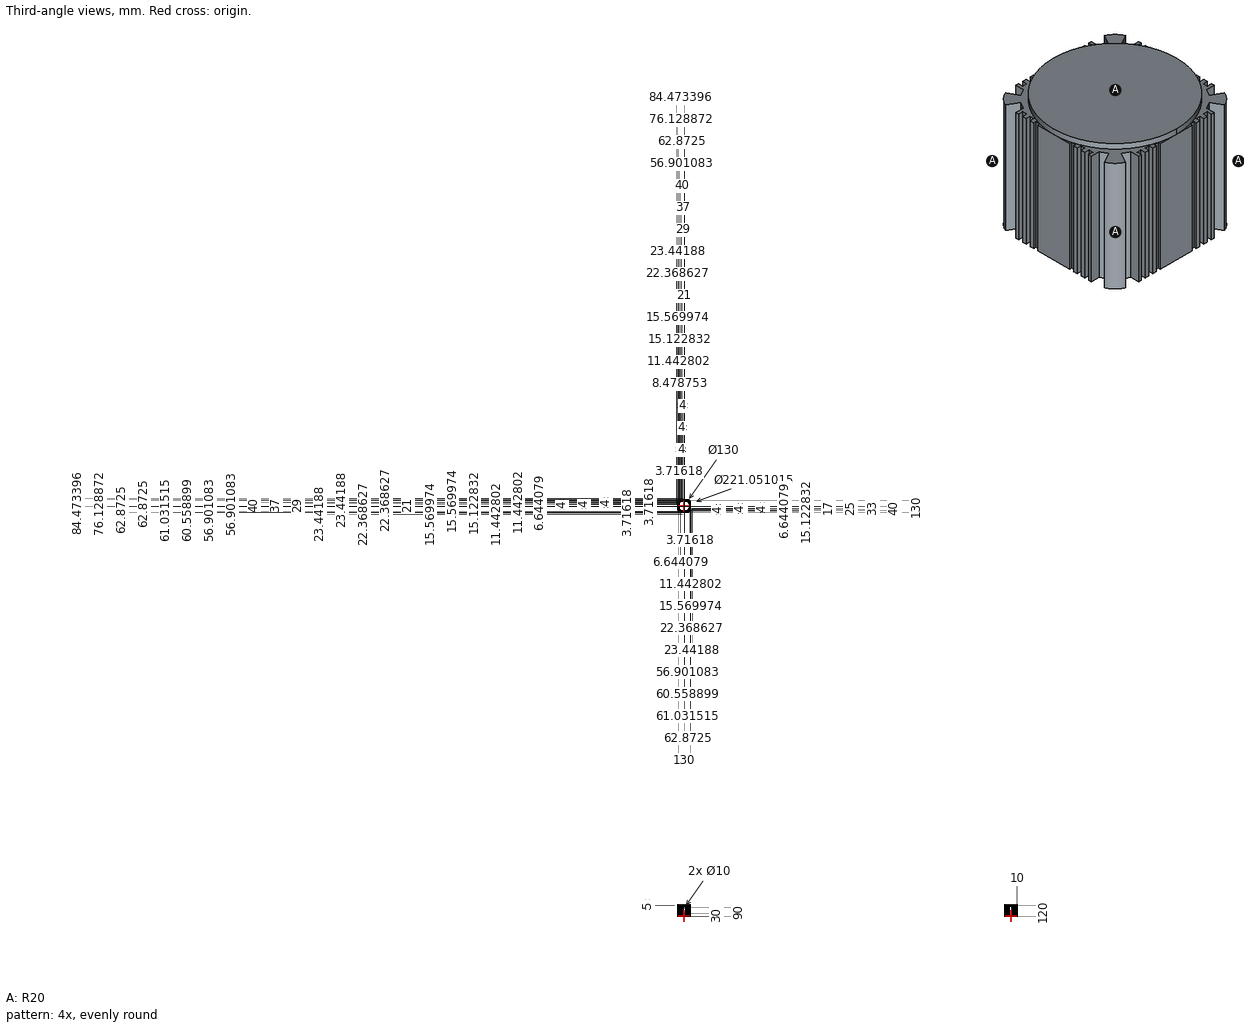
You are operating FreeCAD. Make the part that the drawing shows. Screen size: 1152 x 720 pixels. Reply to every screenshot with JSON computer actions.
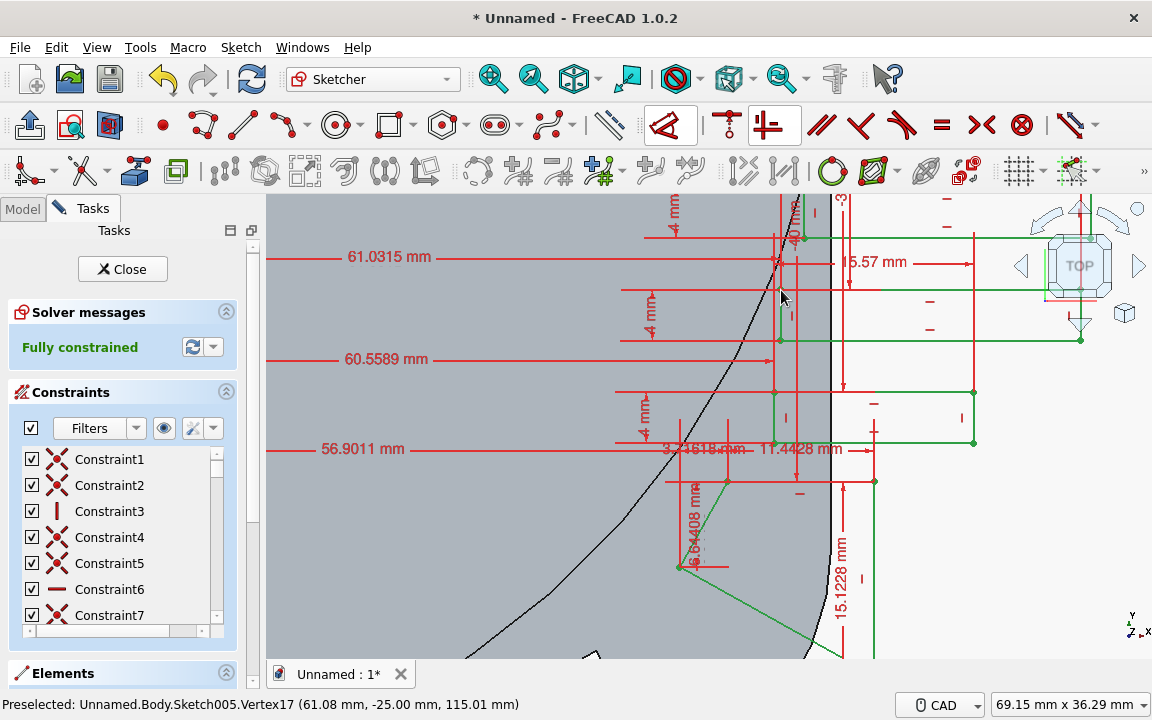
{"action": "left_click", "coordinate": [123, 269]}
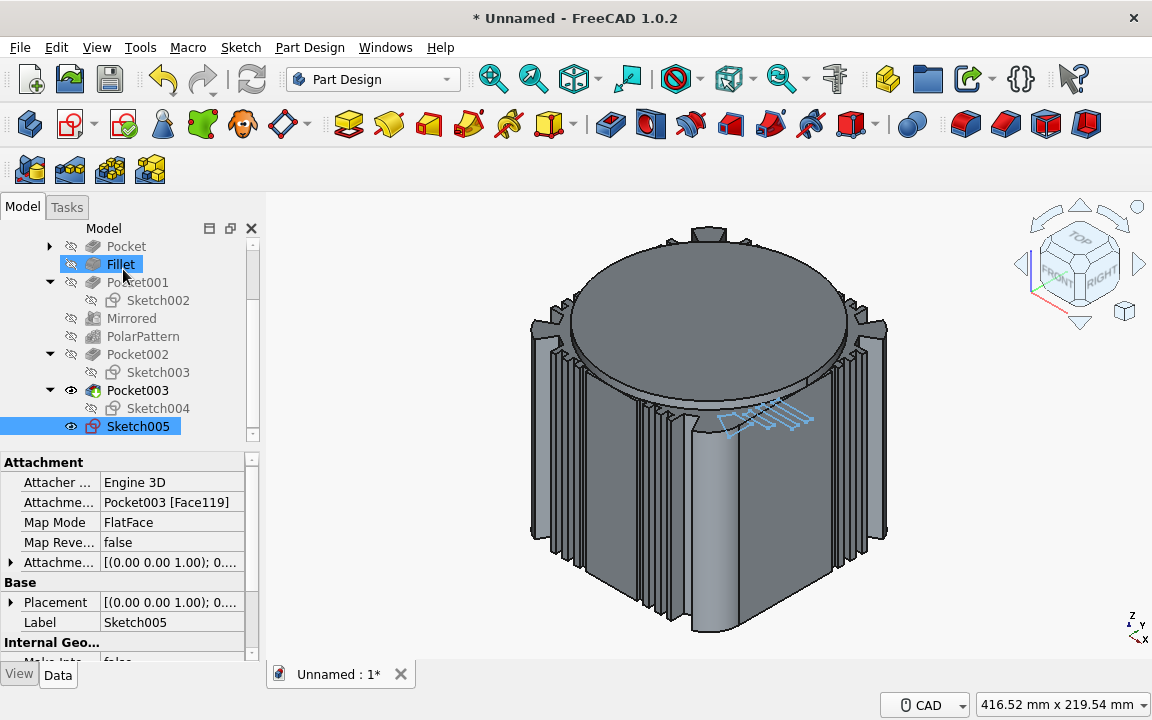
{"action": "left_click", "coordinate": [612, 124]}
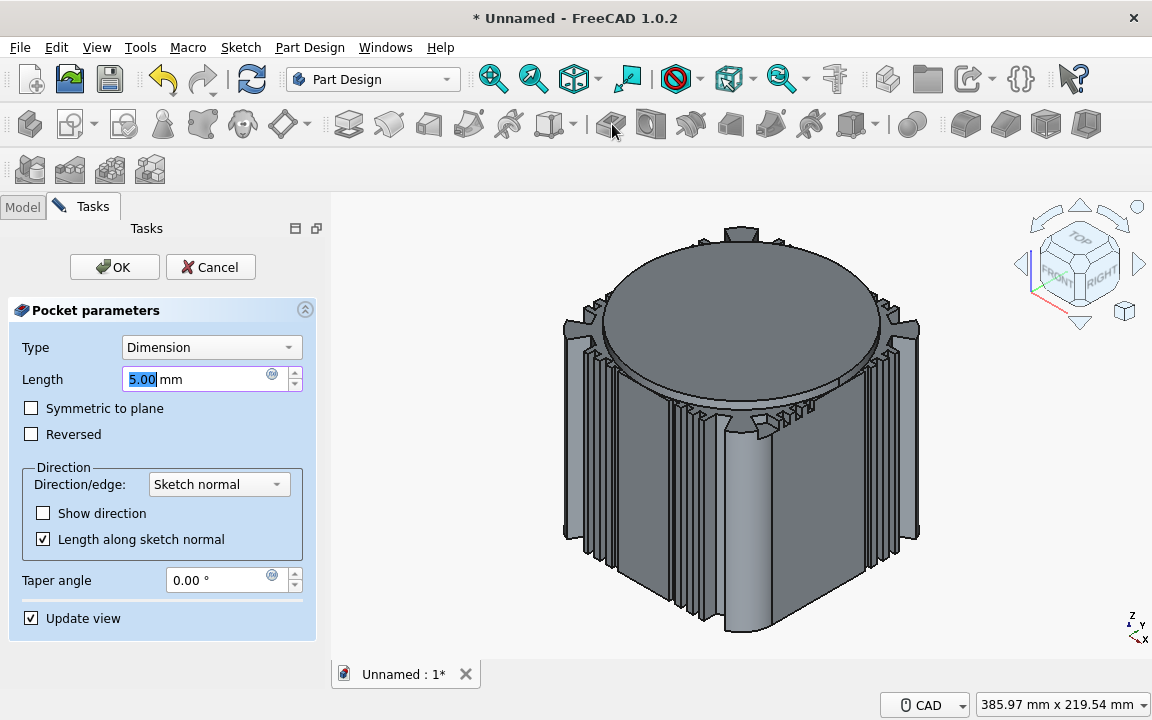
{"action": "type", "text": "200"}
{"action": "key", "text": "Tab"}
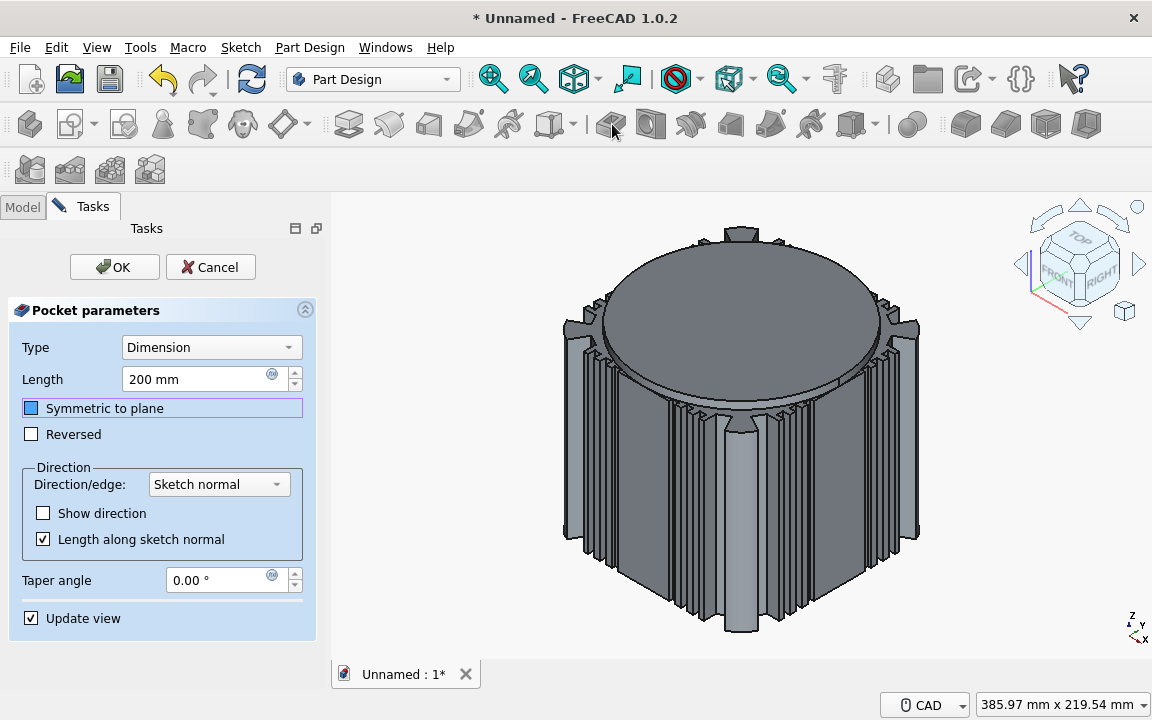
{"action": "left_click", "coordinate": [115, 267]}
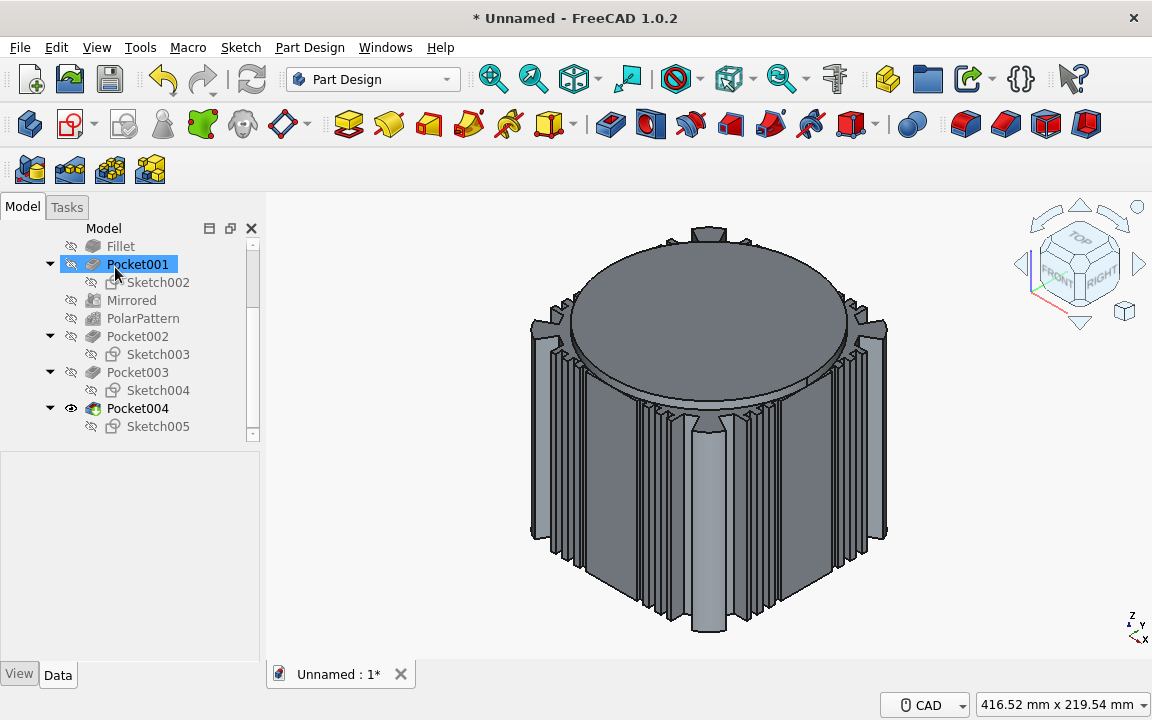
{"action": "key", "text": "4"}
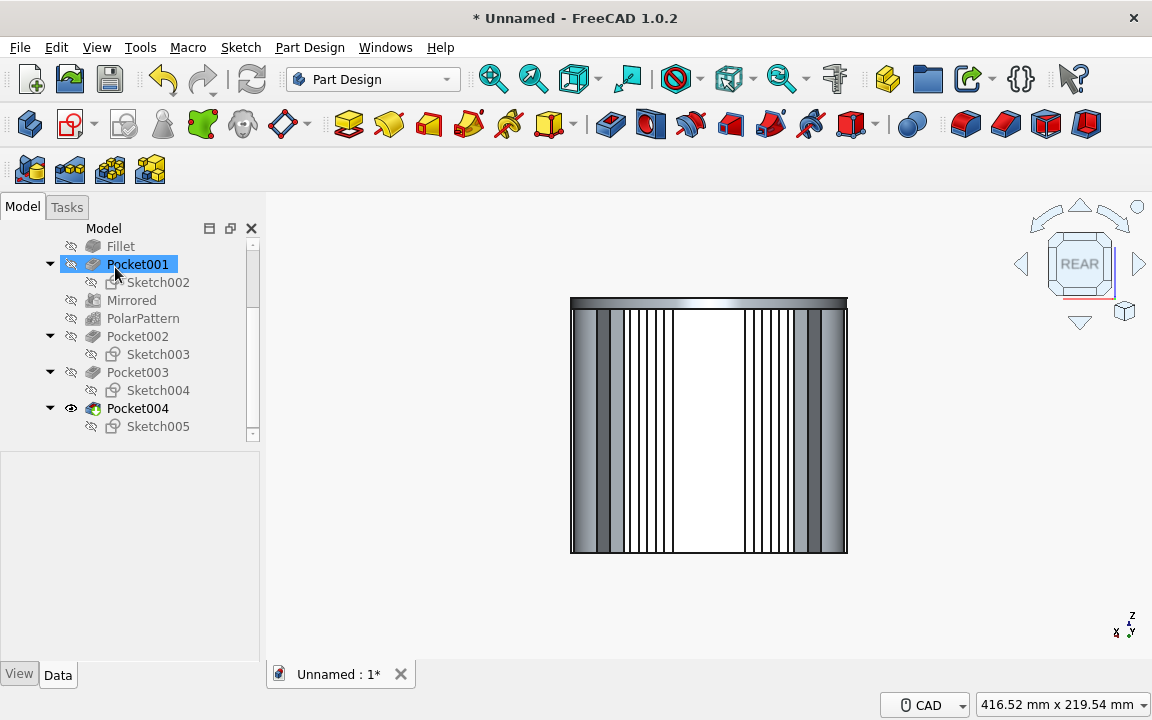
{"action": "left_click", "coordinate": [709, 430]}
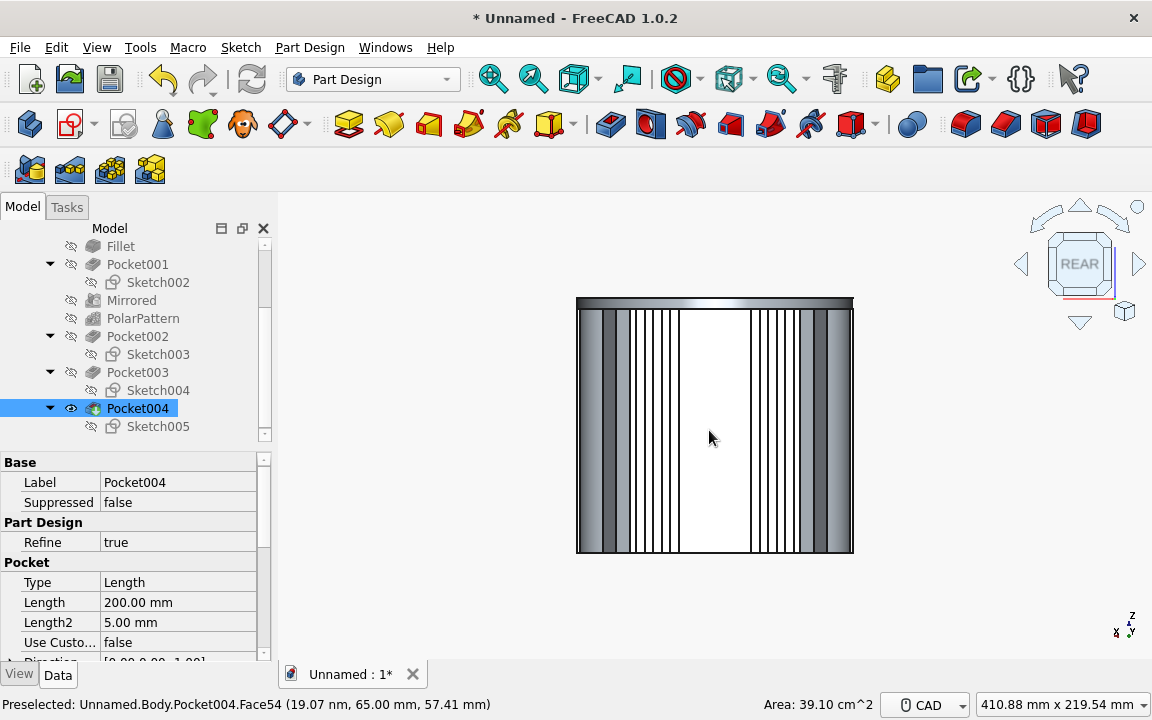
{"action": "left_click", "coordinate": [70, 124]}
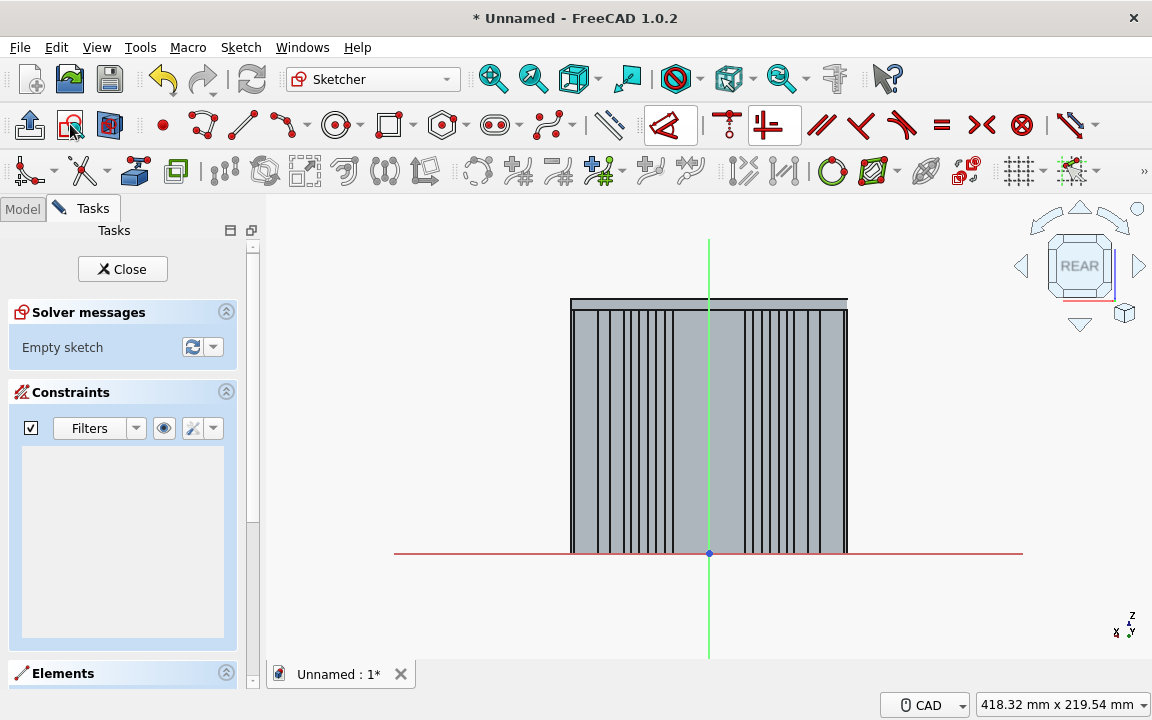
{"action": "scroll", "coordinate": [848, 507], "scroll_direction": "up", "scroll_amount": 2}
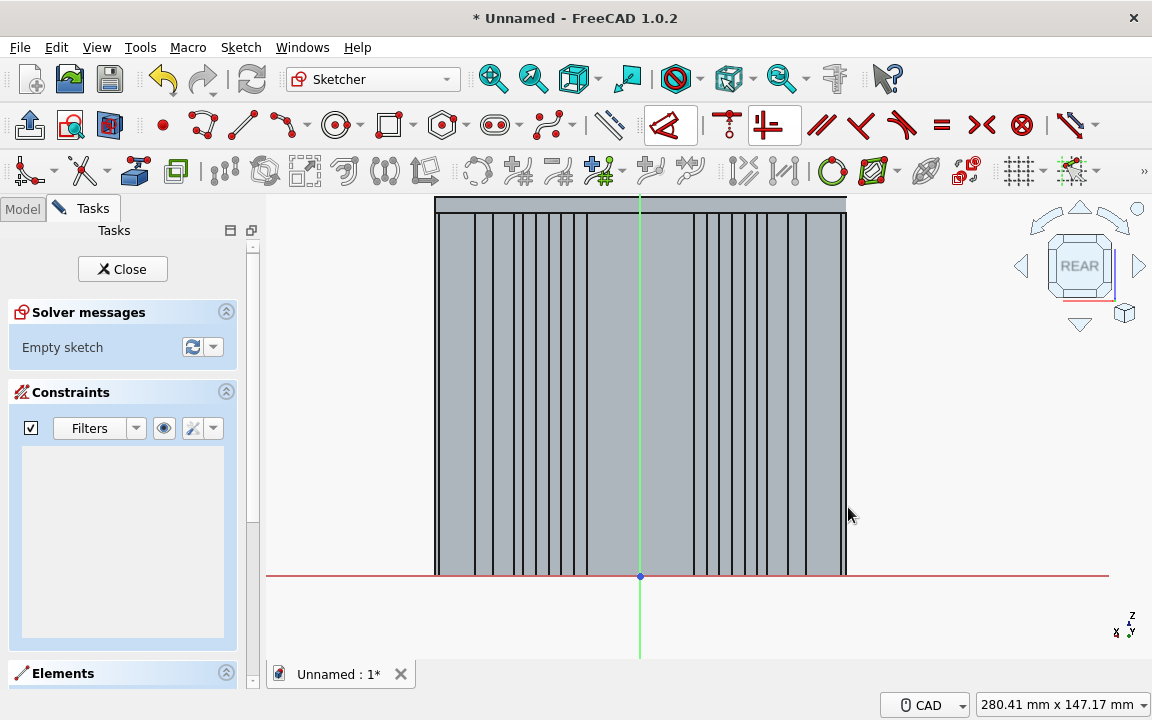
{"action": "left_click", "coordinate": [336, 126]}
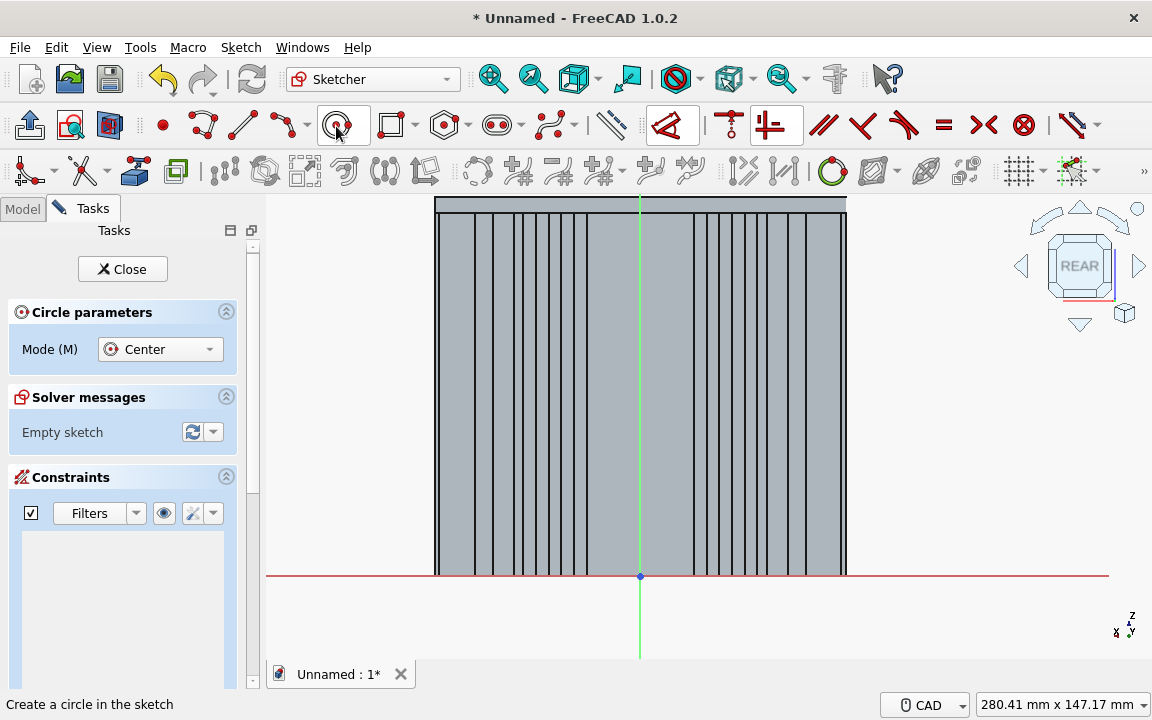
{"action": "scroll", "coordinate": [640, 292], "scroll_direction": "up", "scroll_amount": 2}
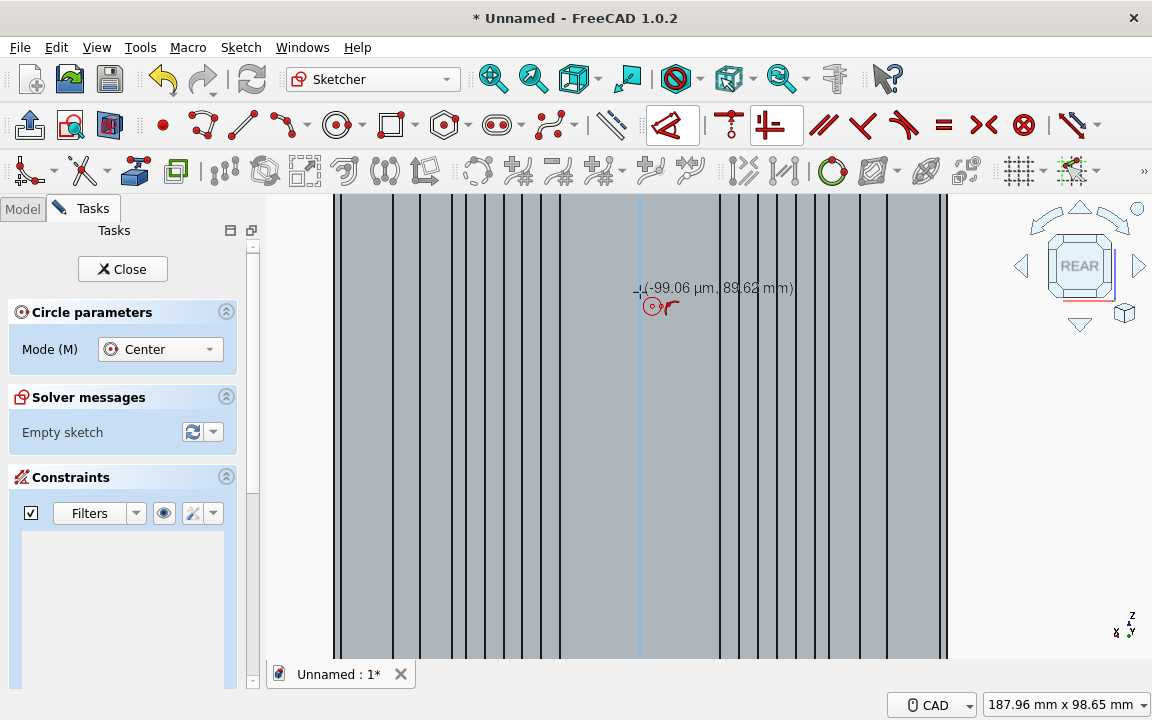
{"action": "left_click", "coordinate": [640, 292]}
{"action": "mouse_move", "coordinate": [657, 275]}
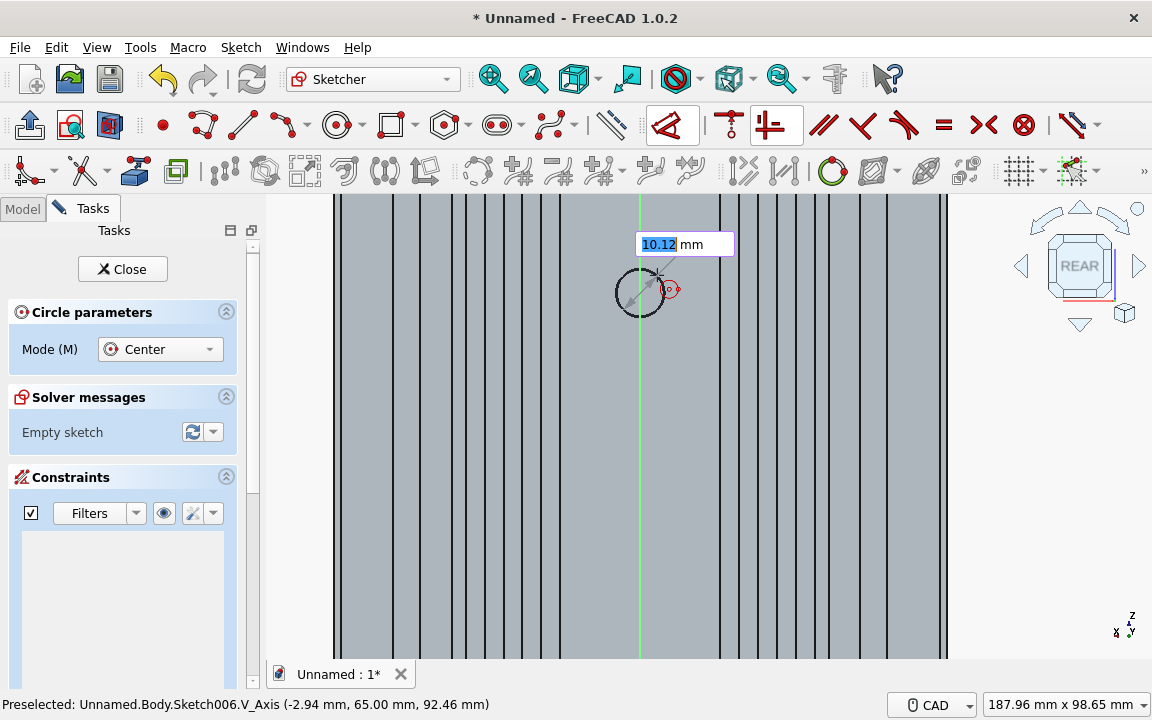
{"action": "type", "text": "10"}
{"action": "key", "text": "Return"}